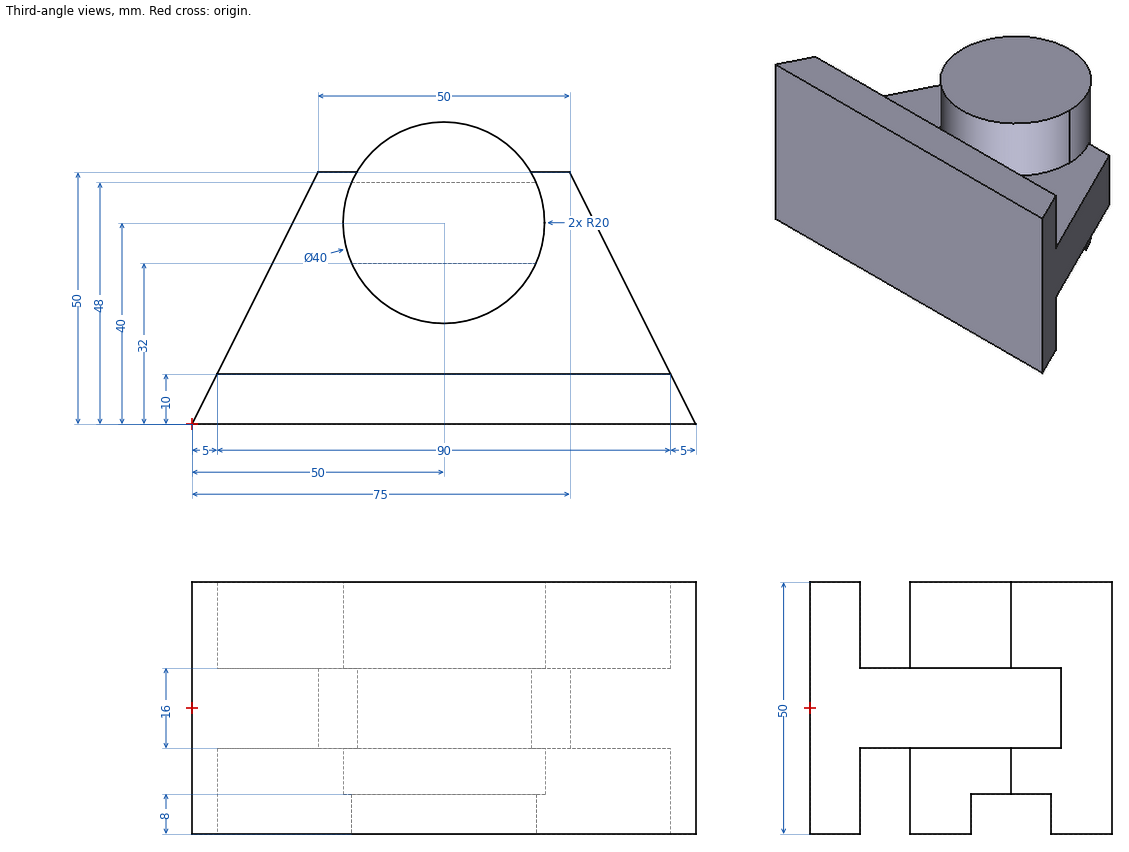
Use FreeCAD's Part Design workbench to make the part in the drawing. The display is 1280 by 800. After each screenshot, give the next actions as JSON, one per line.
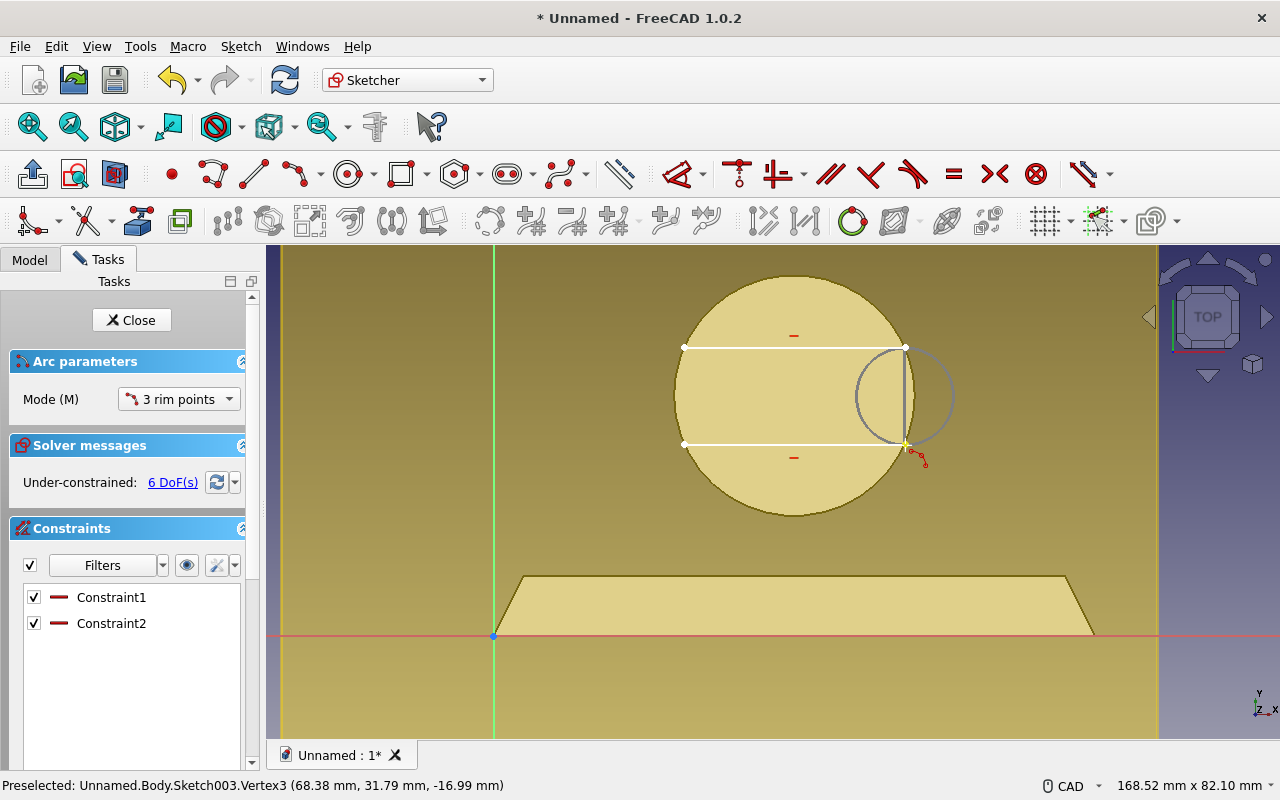
{"action": "scroll", "coordinate": [915, 396], "scroll_direction": "up", "scroll_amount": 3}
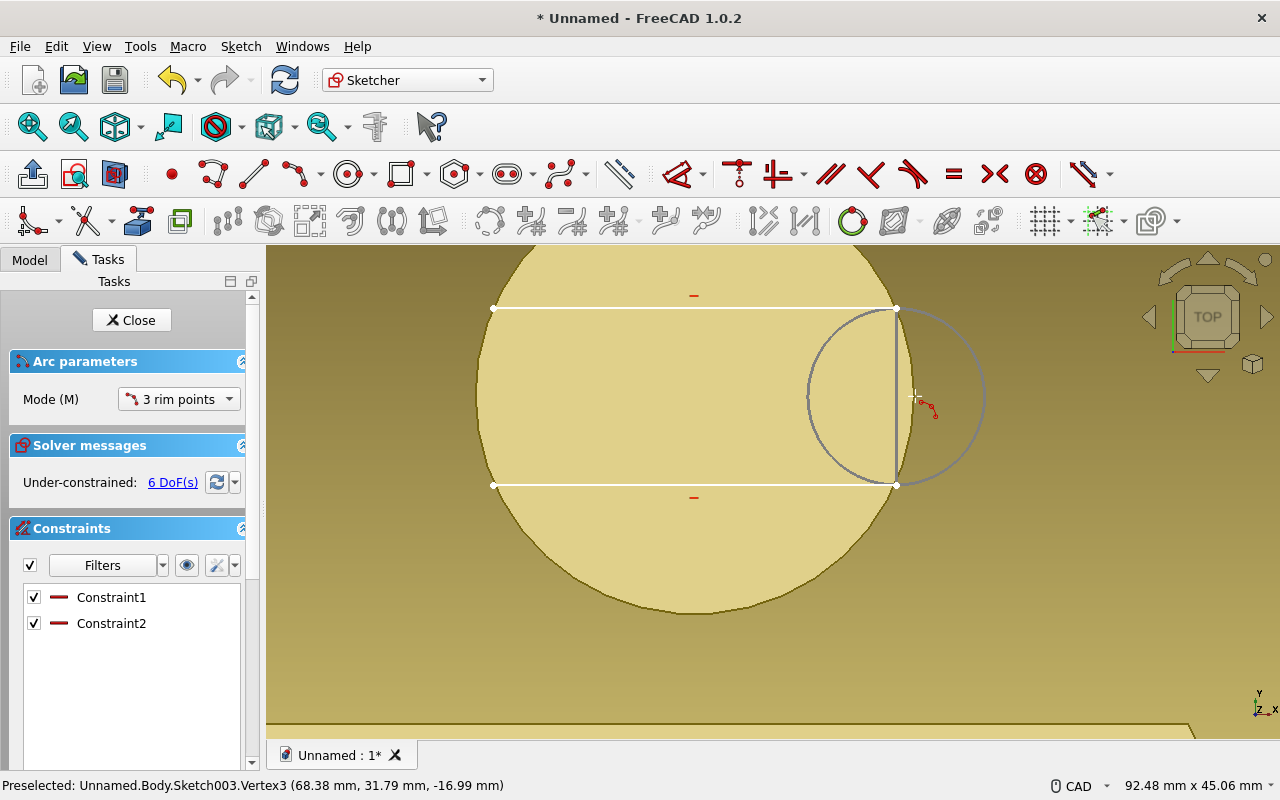
{"action": "left_click", "coordinate": [914, 395]}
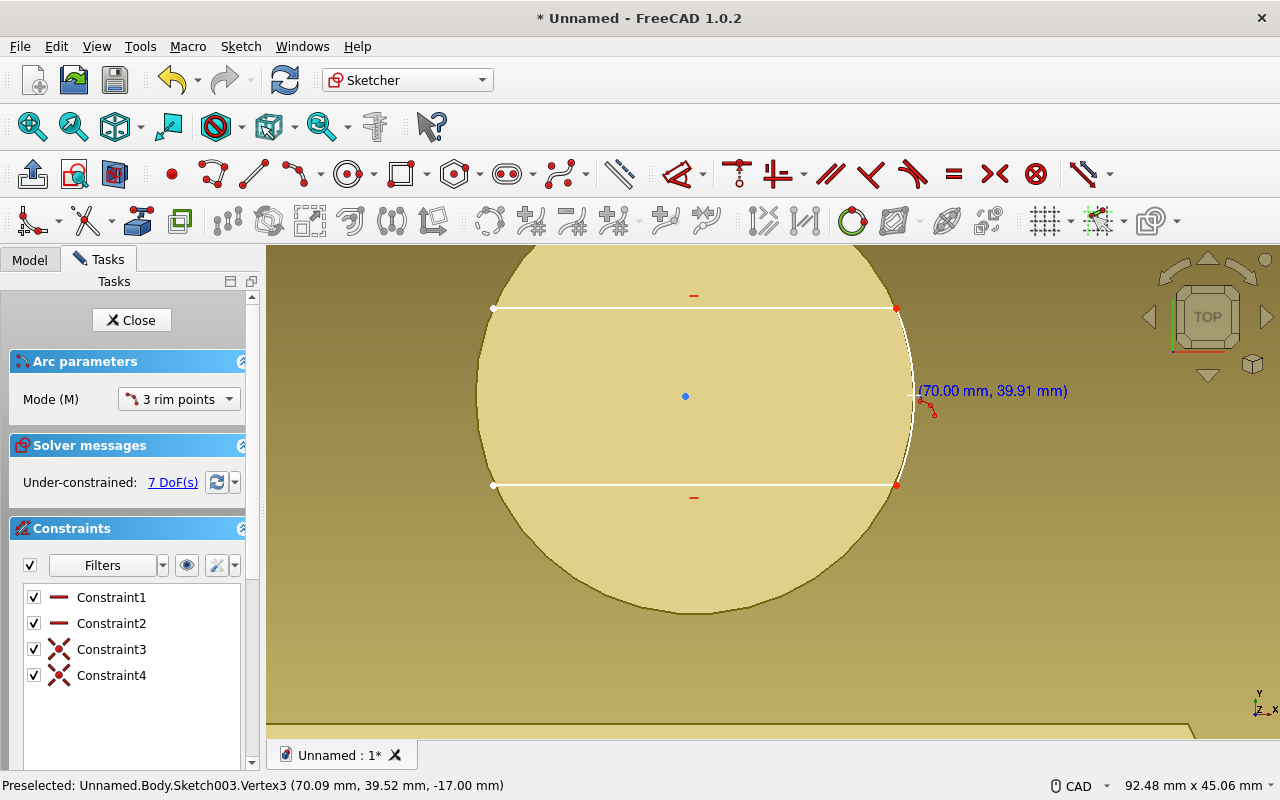
{"action": "left_click", "coordinate": [494, 485]}
{"action": "left_click", "coordinate": [494, 308]}
{"action": "left_click", "coordinate": [475, 395]}
{"action": "key", "text": "Escape"}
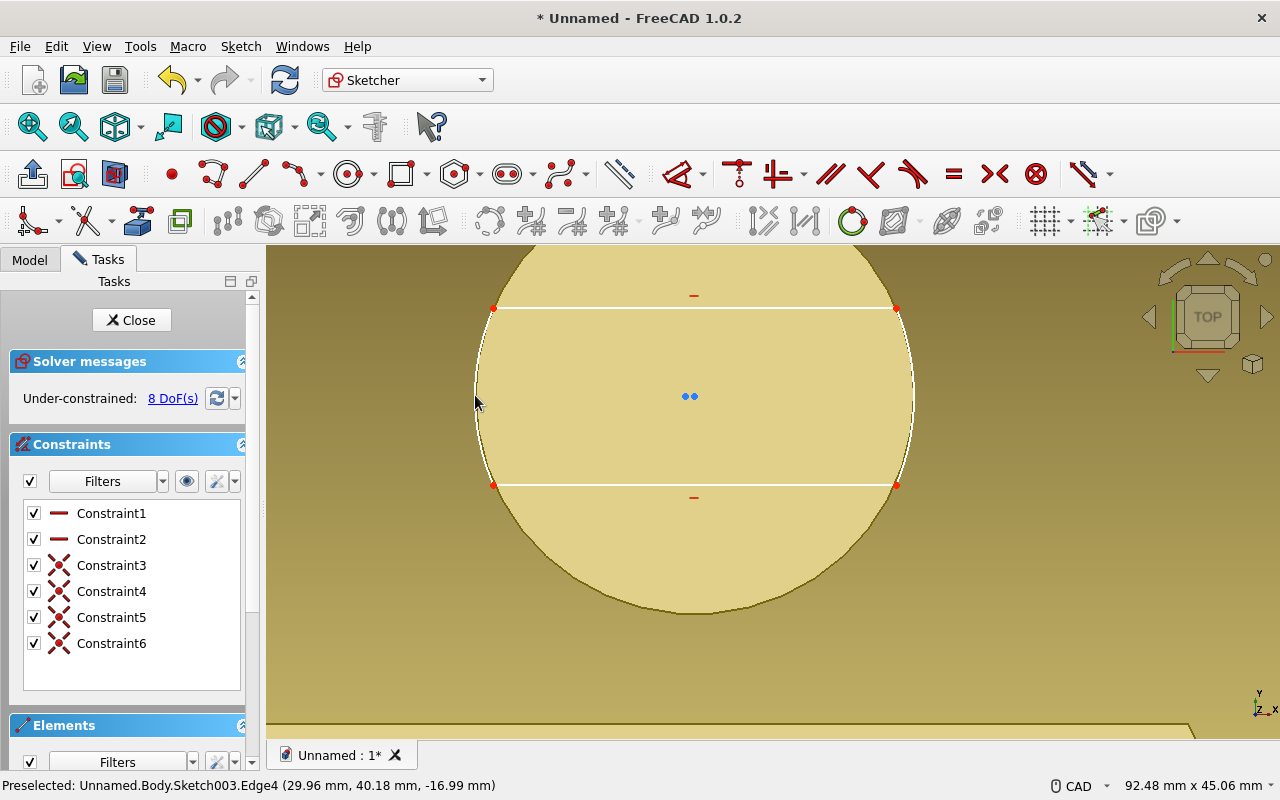
{"action": "left_click", "coordinate": [911, 433]}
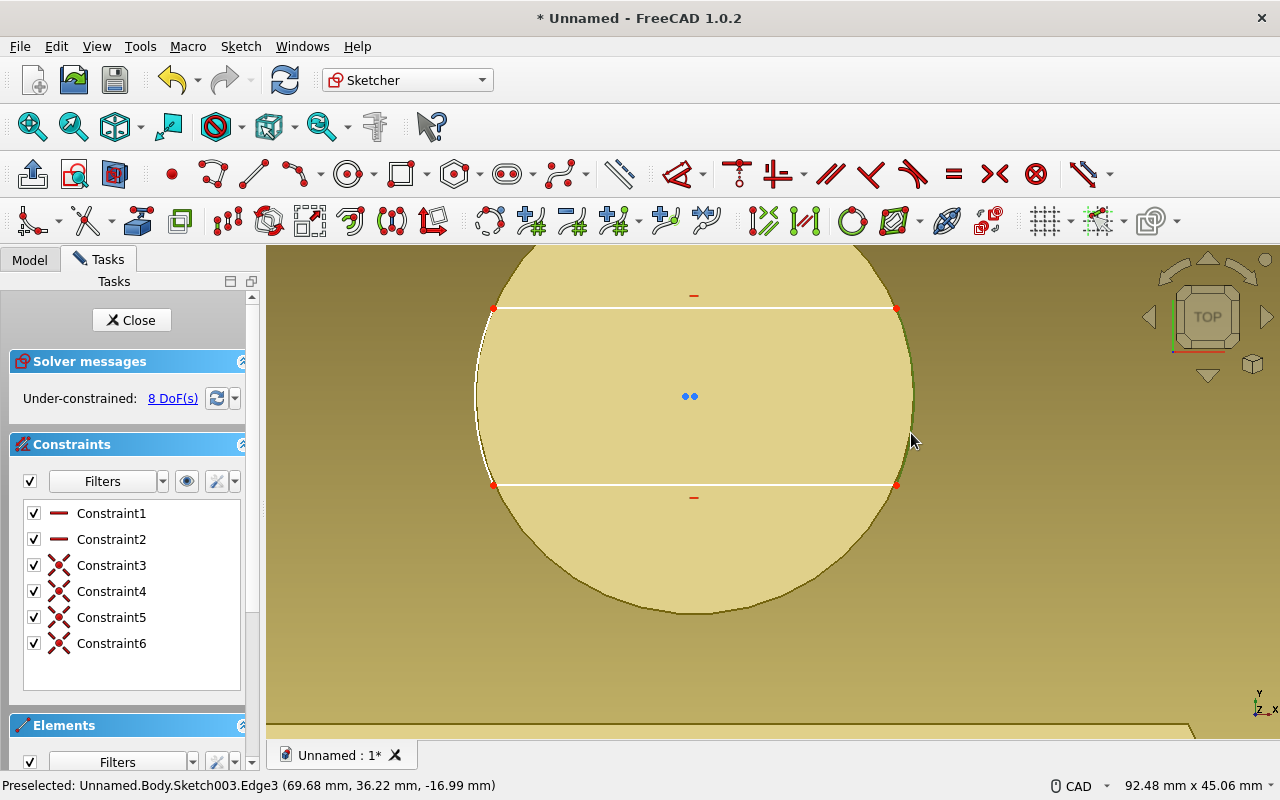
{"action": "left_click", "coordinate": [478, 360]}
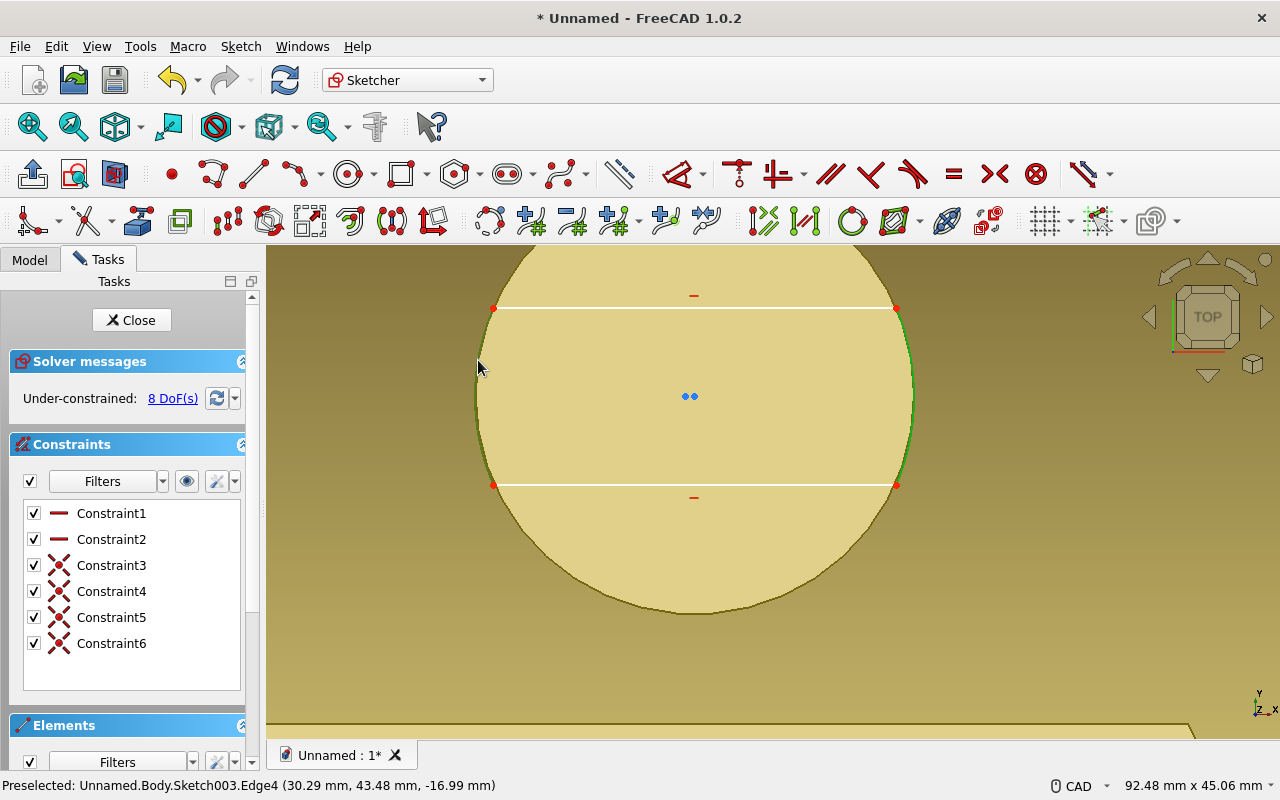
{"action": "left_click", "coordinate": [737, 174]}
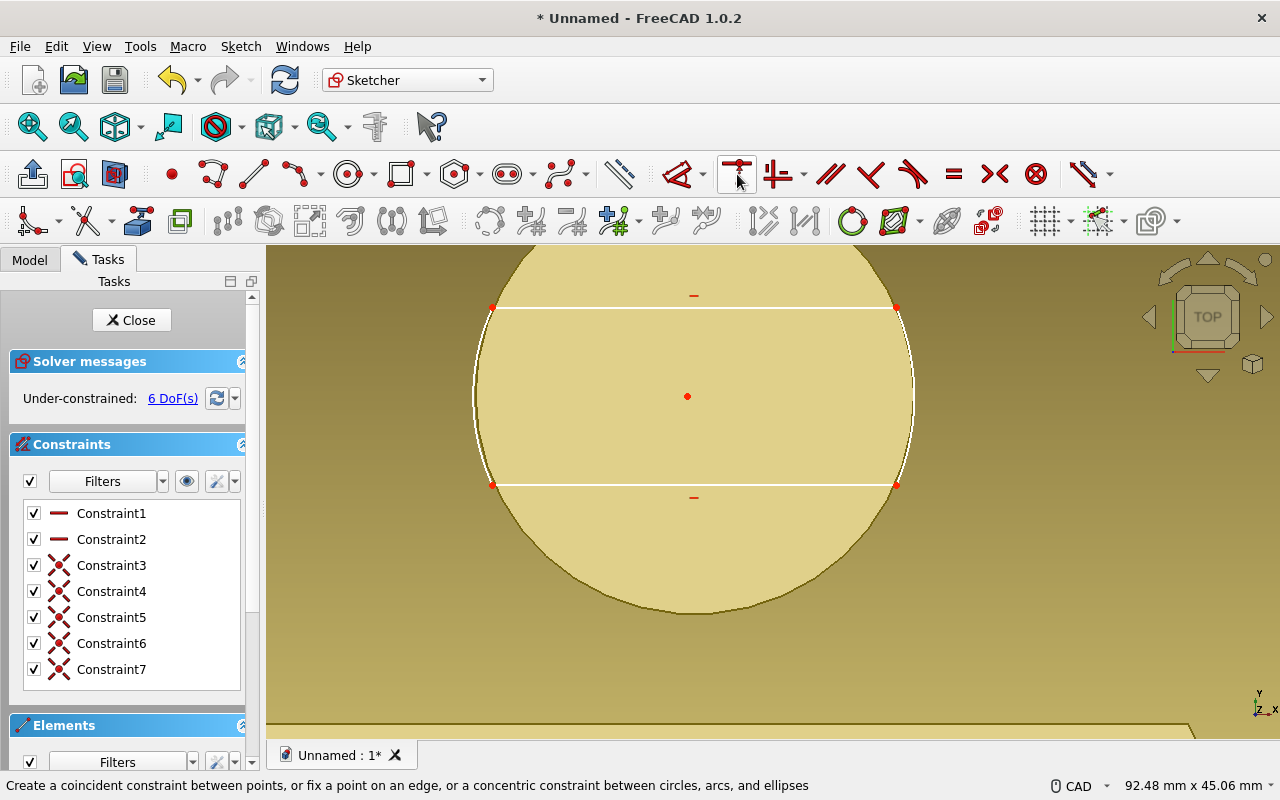
{"action": "left_click", "coordinate": [911, 433]}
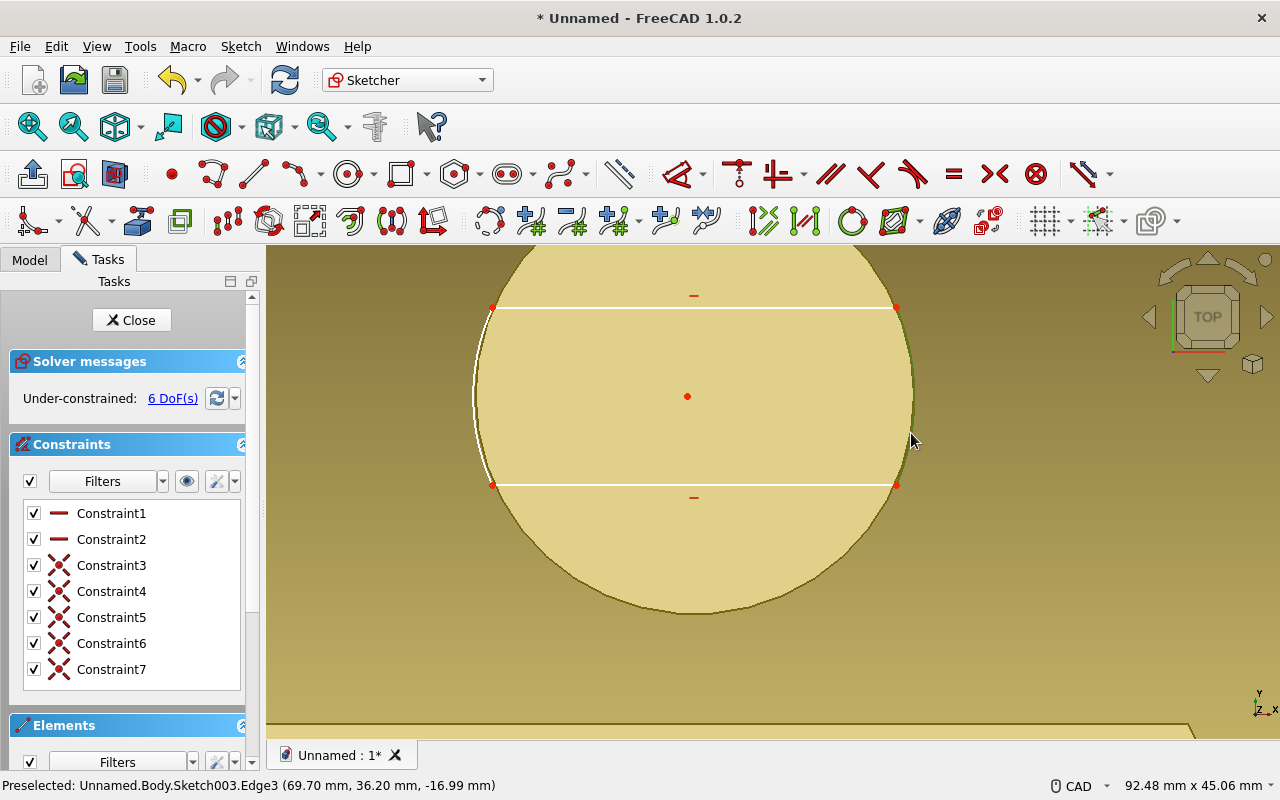
{"action": "left_click", "coordinate": [476, 360]}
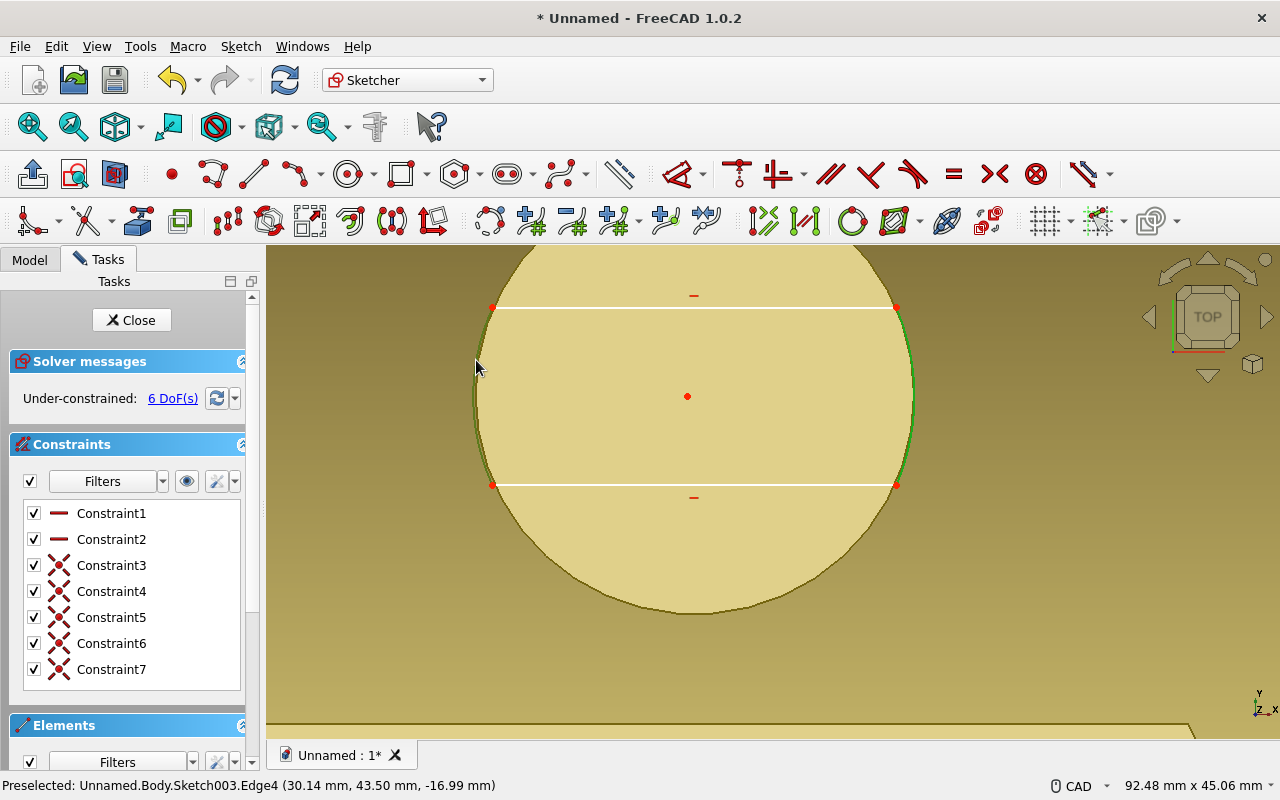
{"action": "left_click", "coordinate": [954, 174]}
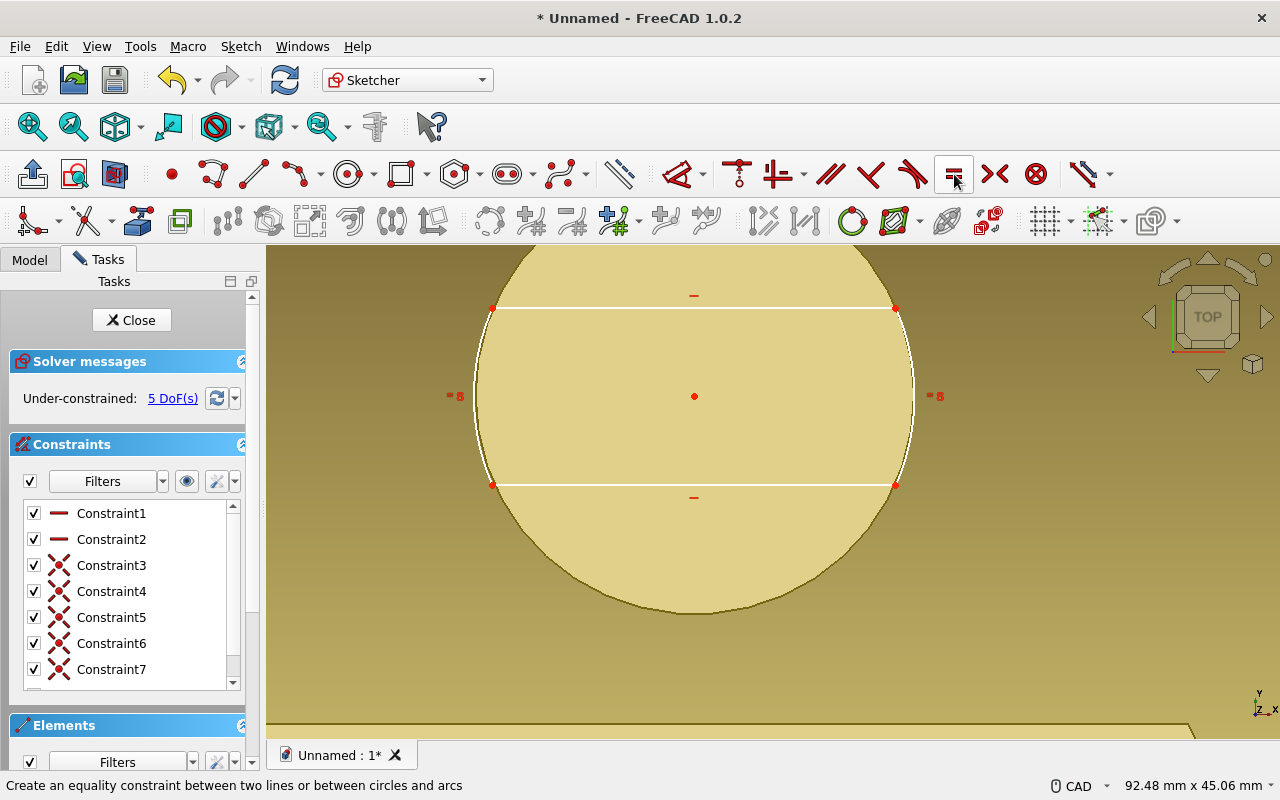
{"action": "left_click", "coordinate": [676, 174]}